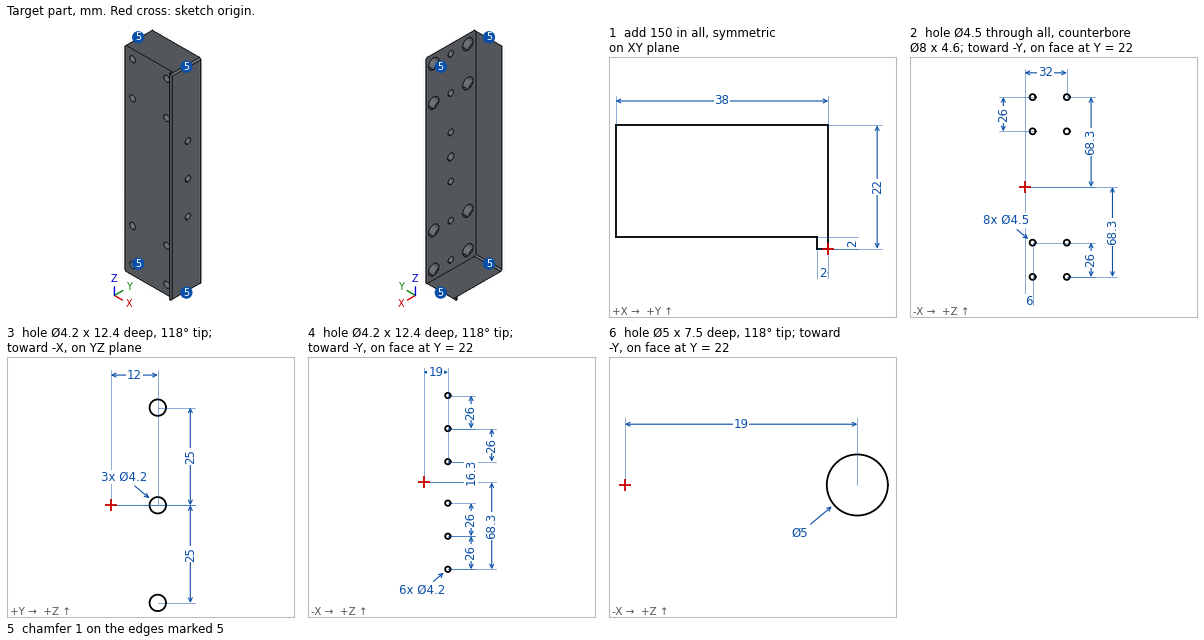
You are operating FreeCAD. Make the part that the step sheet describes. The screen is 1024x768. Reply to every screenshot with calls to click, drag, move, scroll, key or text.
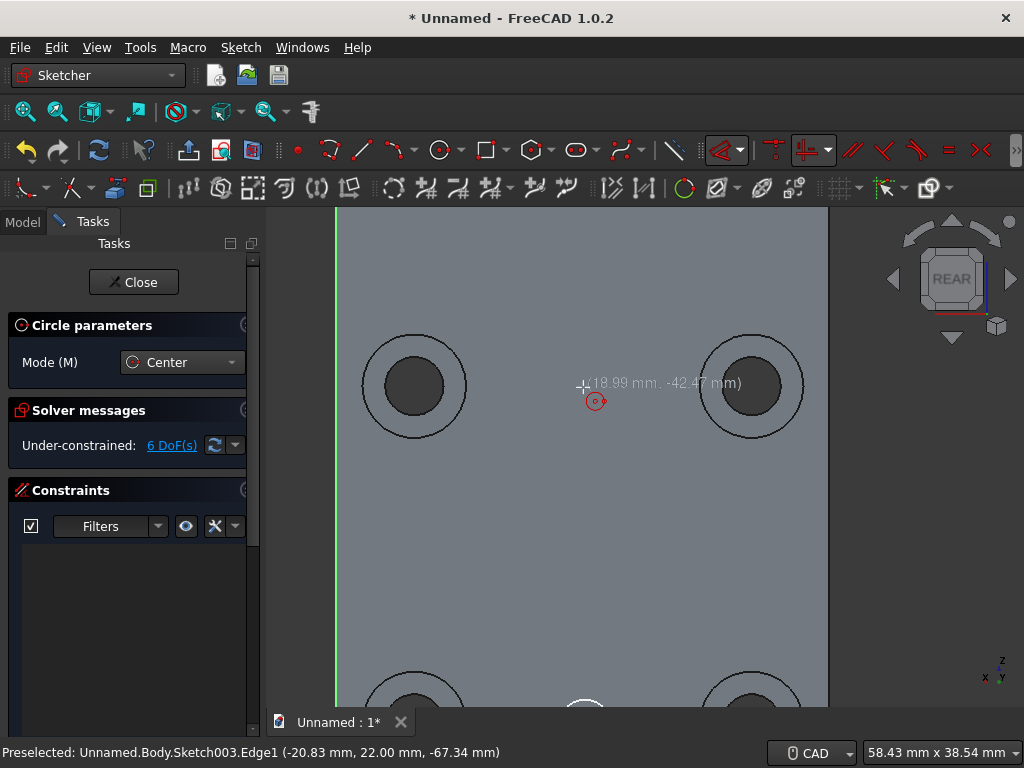
scroll(597, 580, down, 9)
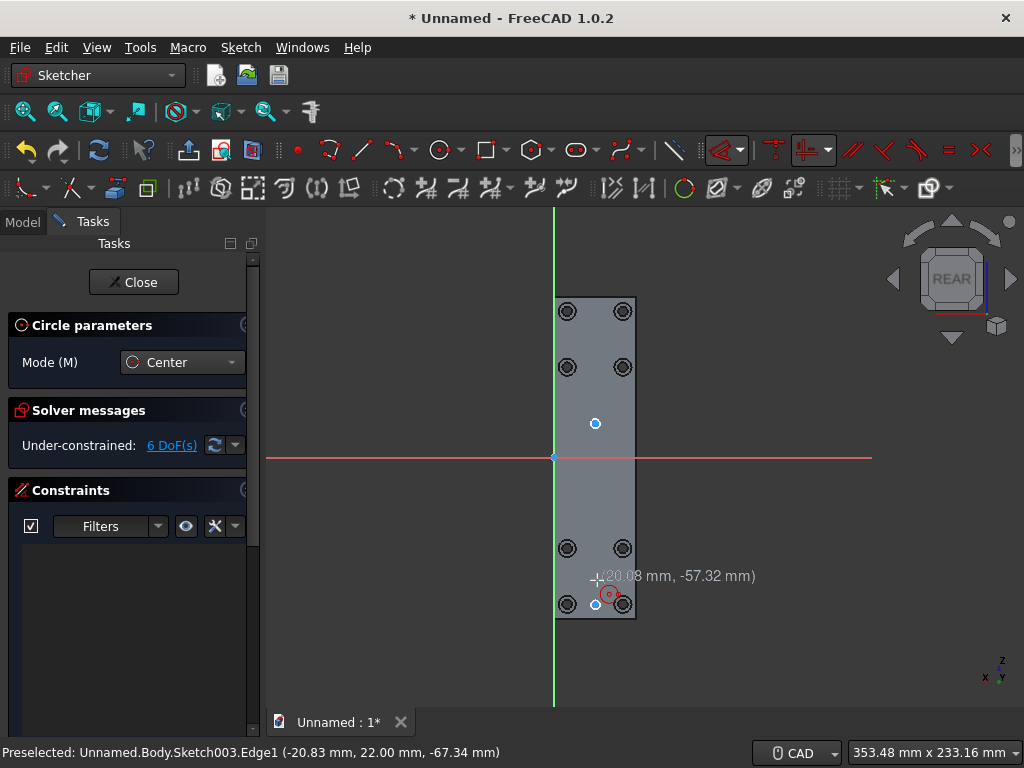
click(595, 549)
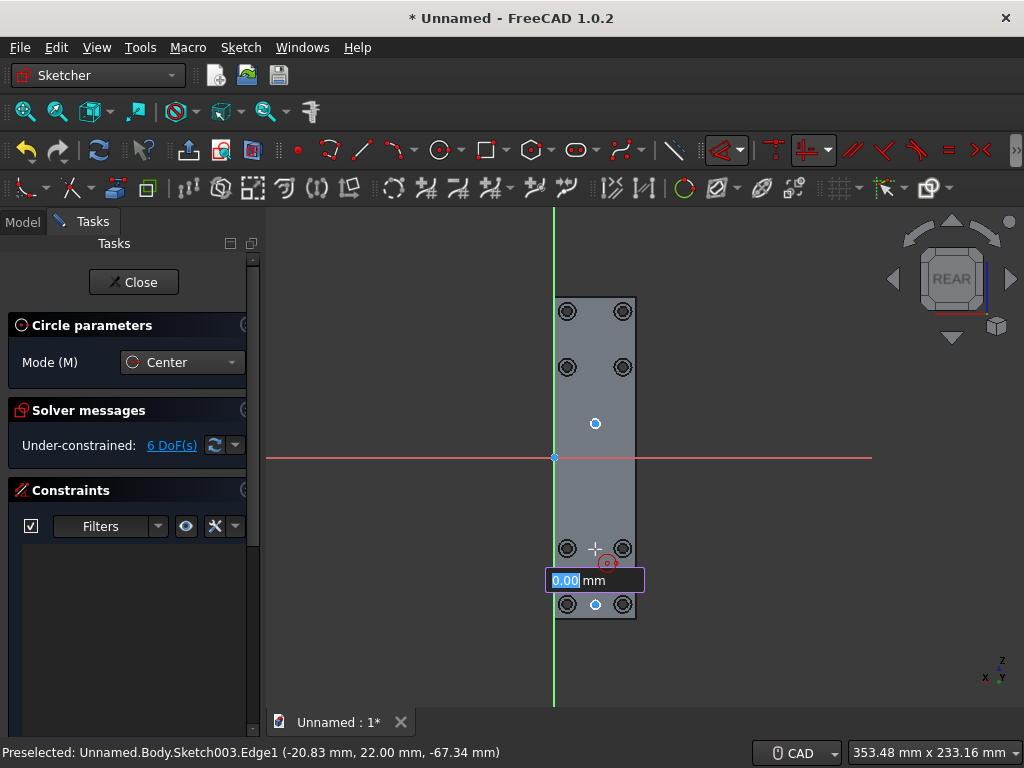
scroll(598, 545, up, 7)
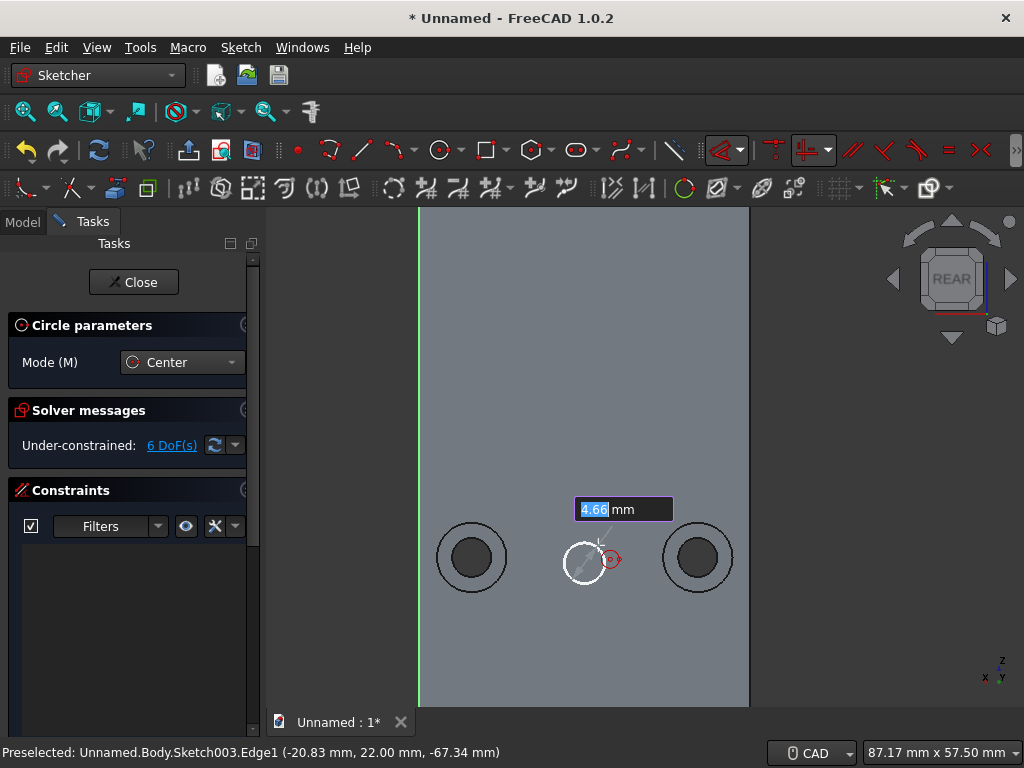
click(598, 545)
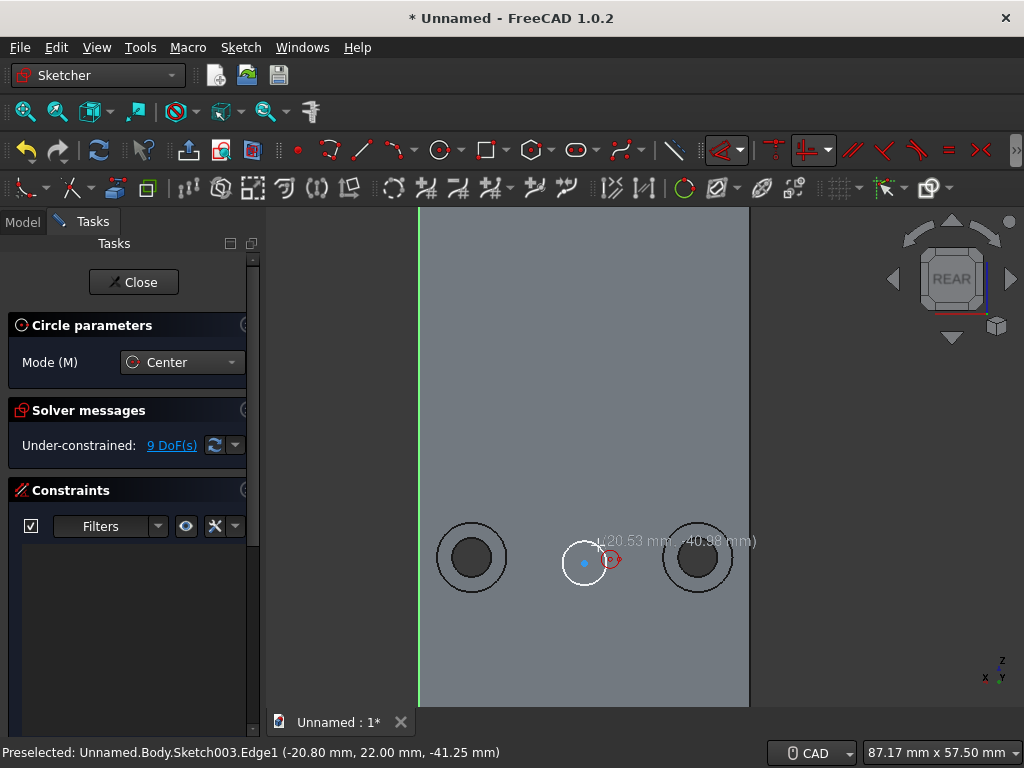
scroll(598, 545, down, 7)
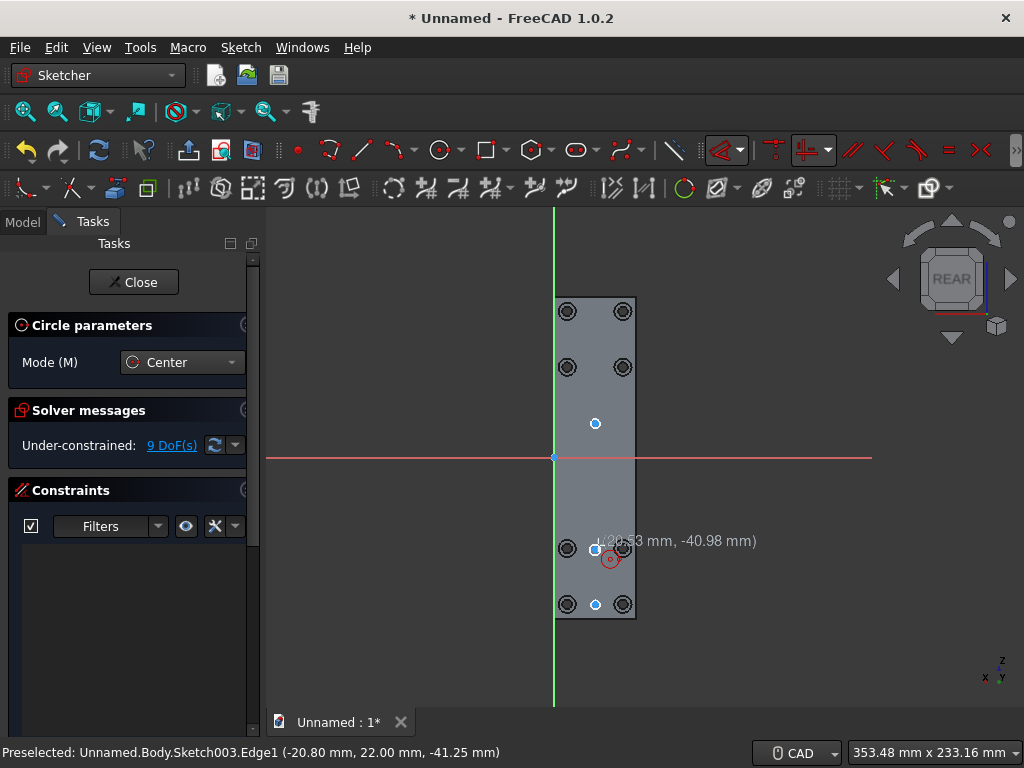
scroll(595, 367, up, 9)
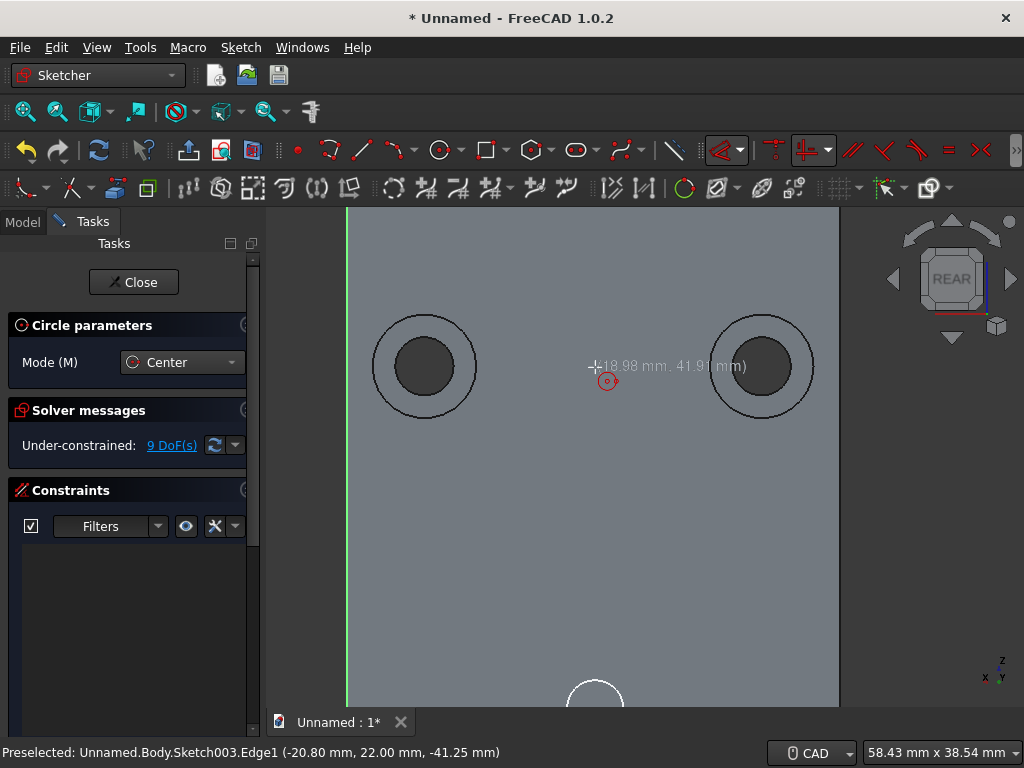
scroll(595, 366, down, 9)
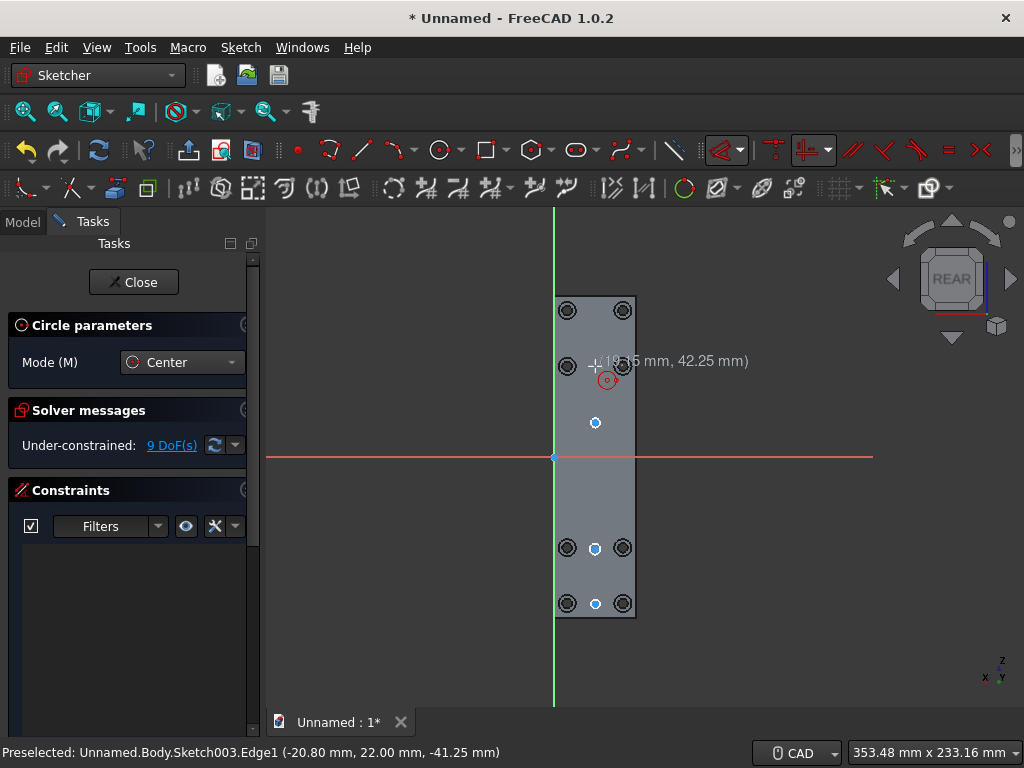
click(595, 366)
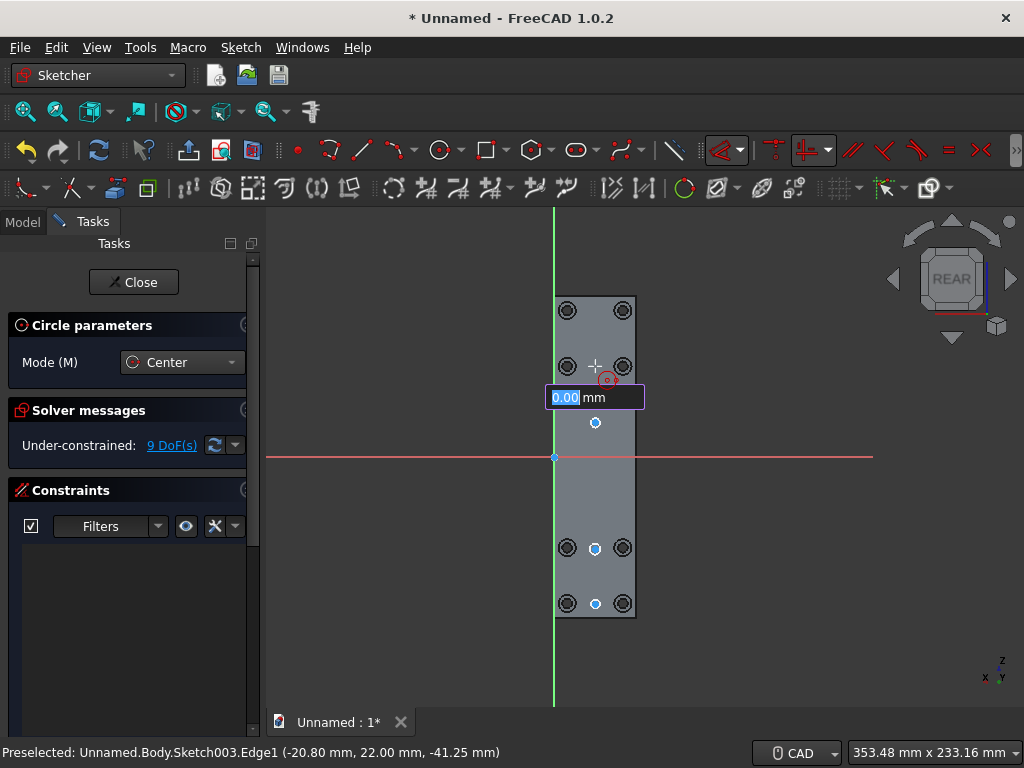
scroll(598, 363, up, 7)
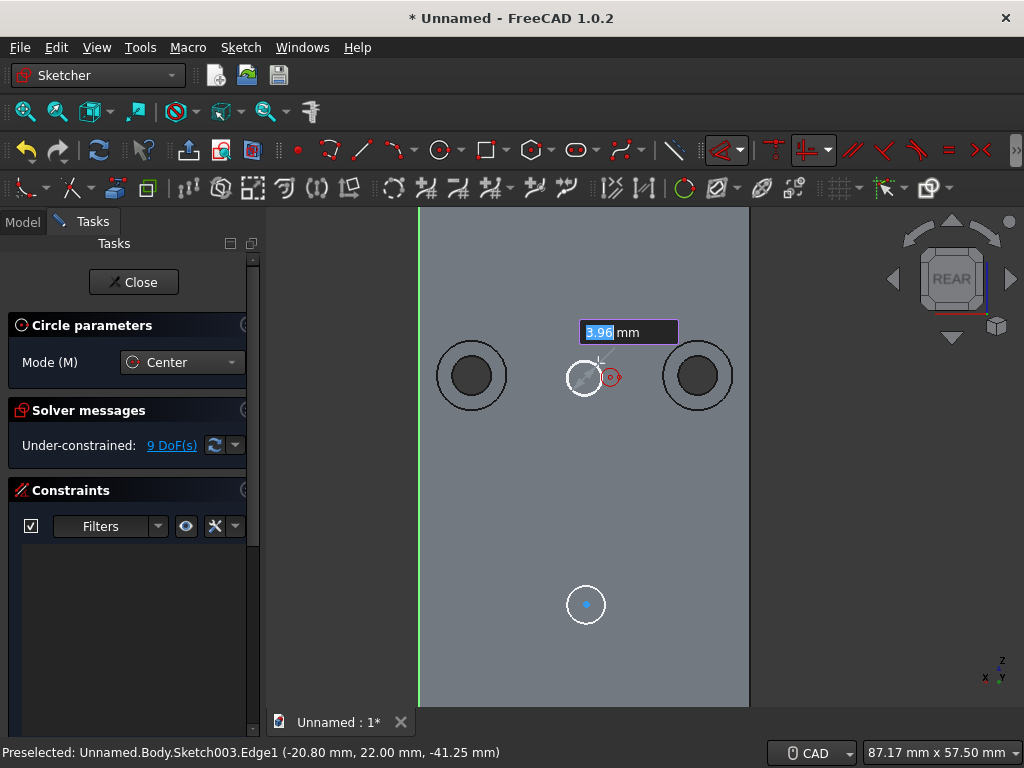
click(598, 363)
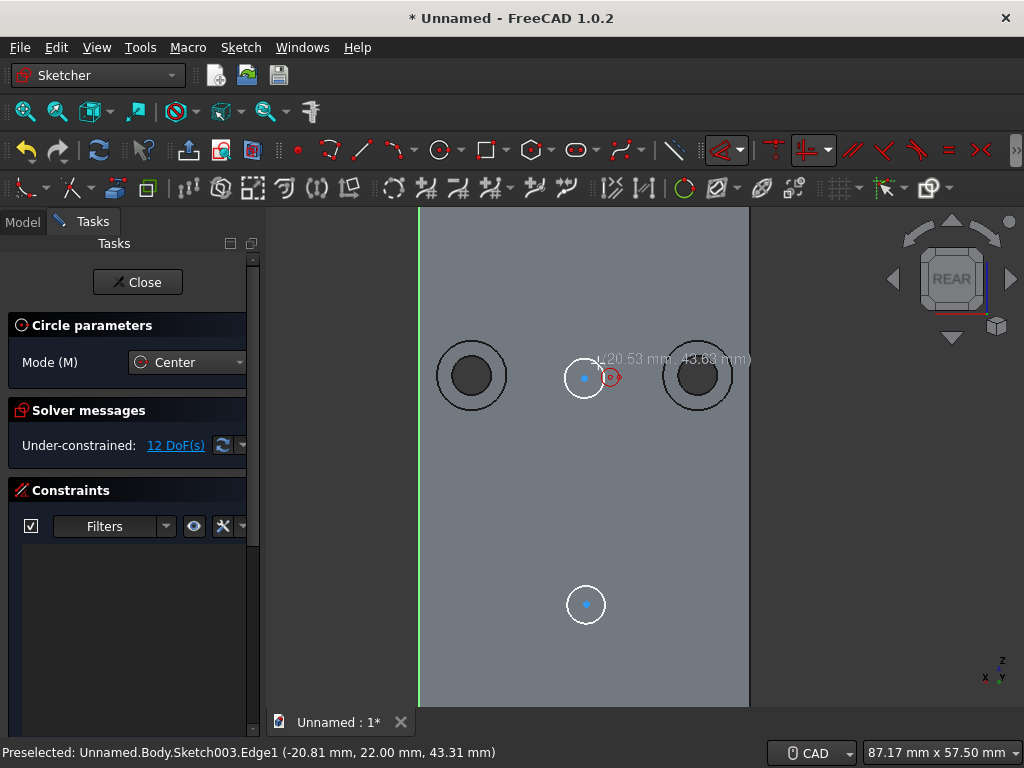
scroll(598, 363, down, 7)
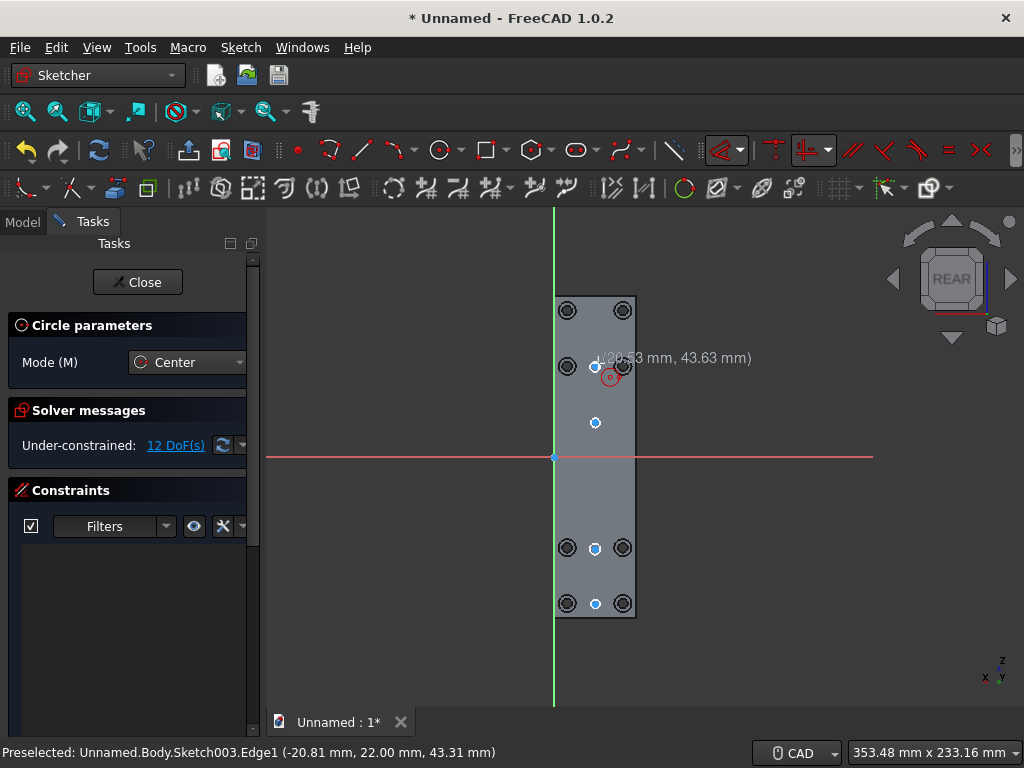
scroll(595, 311, up, 9)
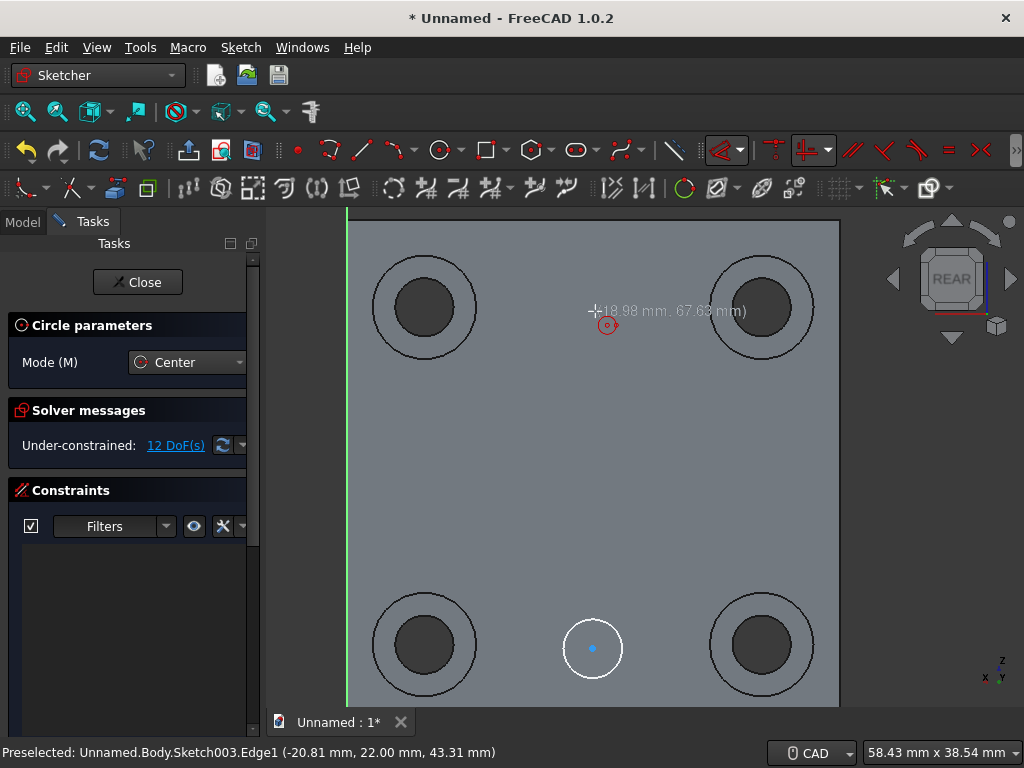
scroll(595, 311, down, 9)